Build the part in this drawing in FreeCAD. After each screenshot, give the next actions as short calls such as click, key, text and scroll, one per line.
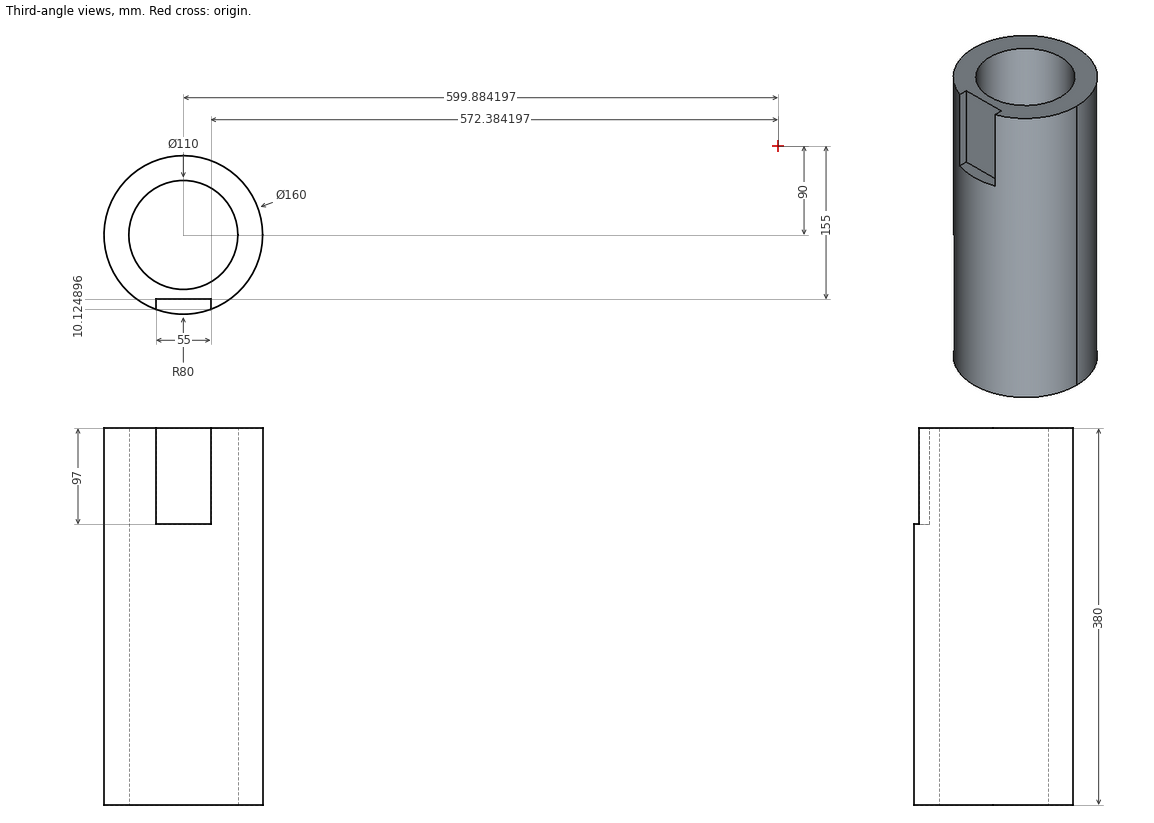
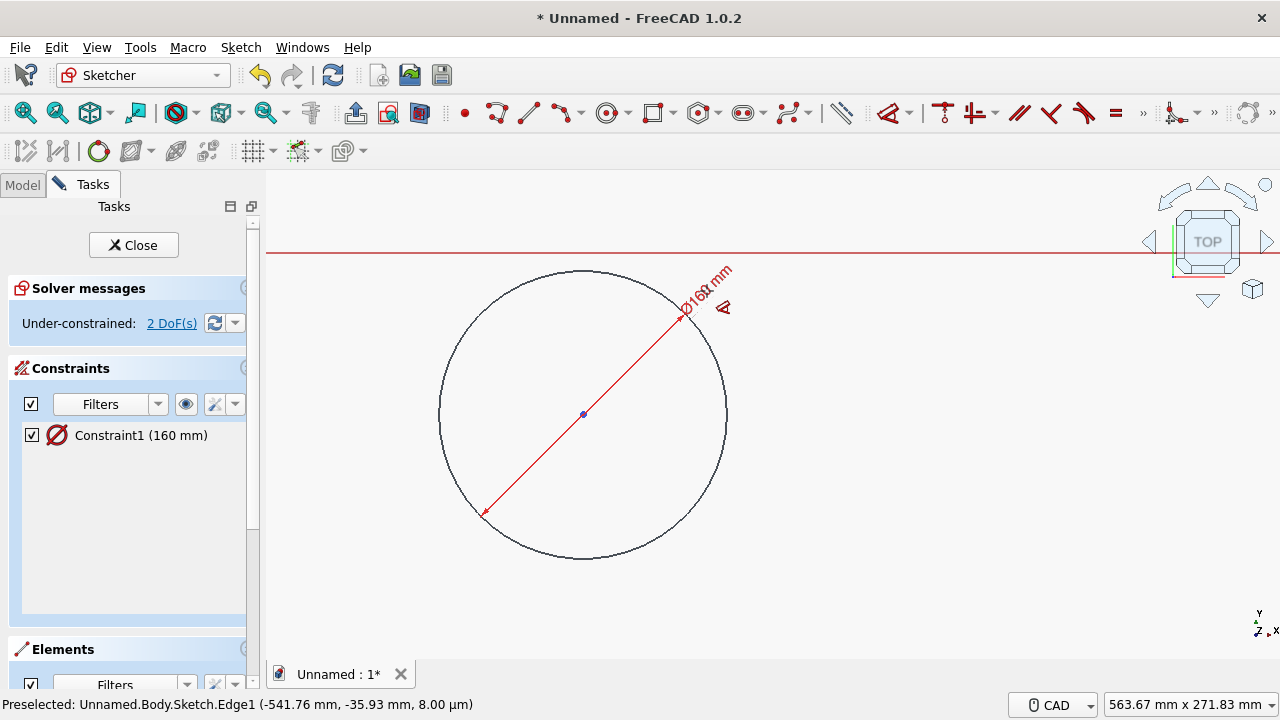
click(583, 415)
click(549, 334)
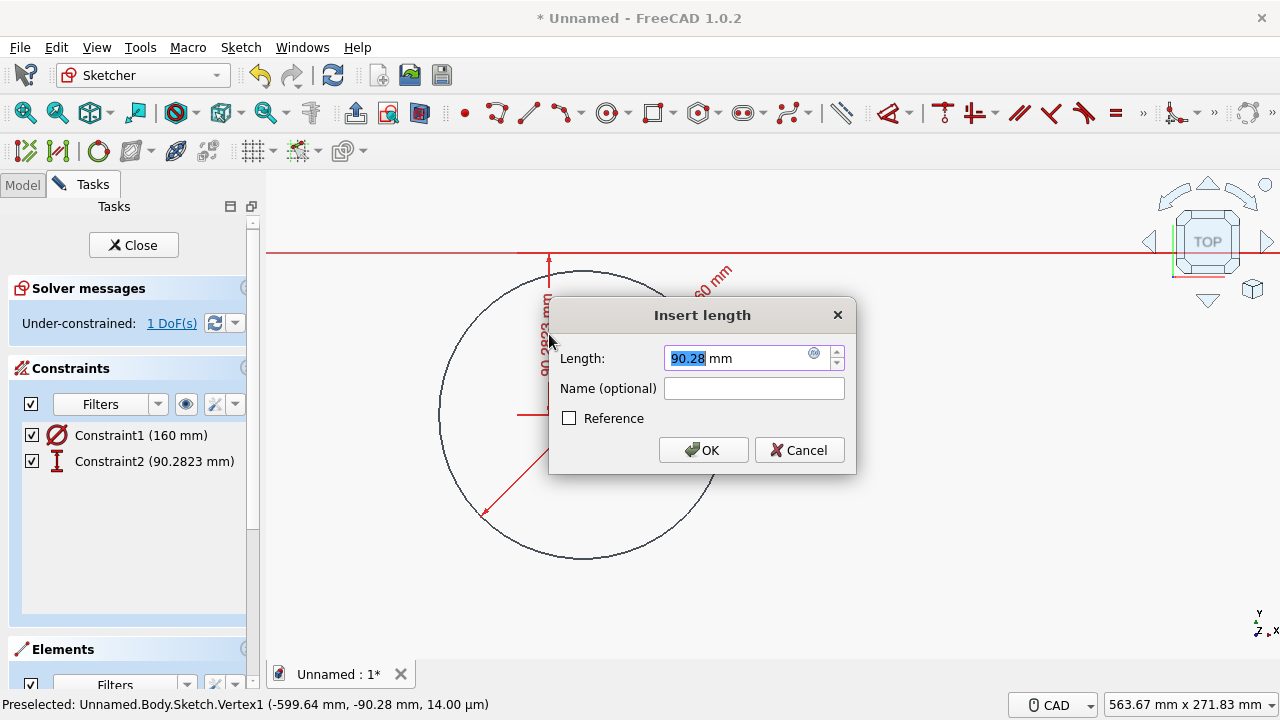
text(90)
key(Return)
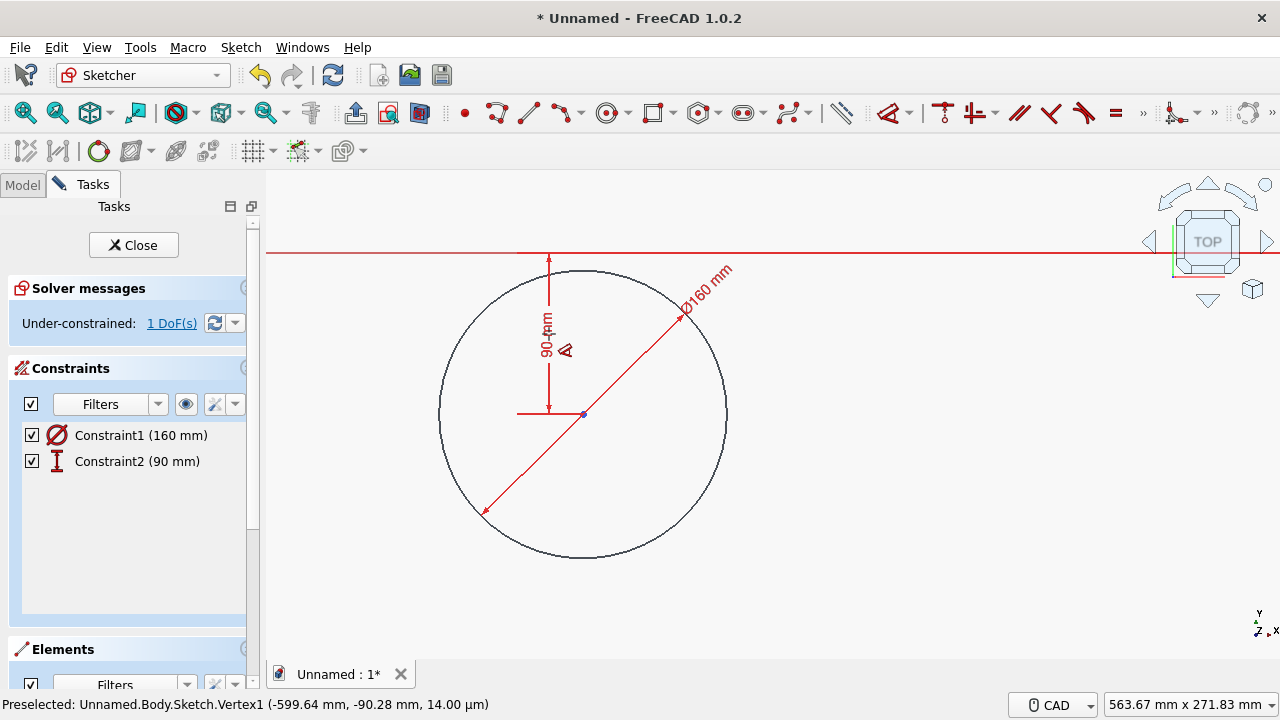
click(583, 414)
click(849, 219)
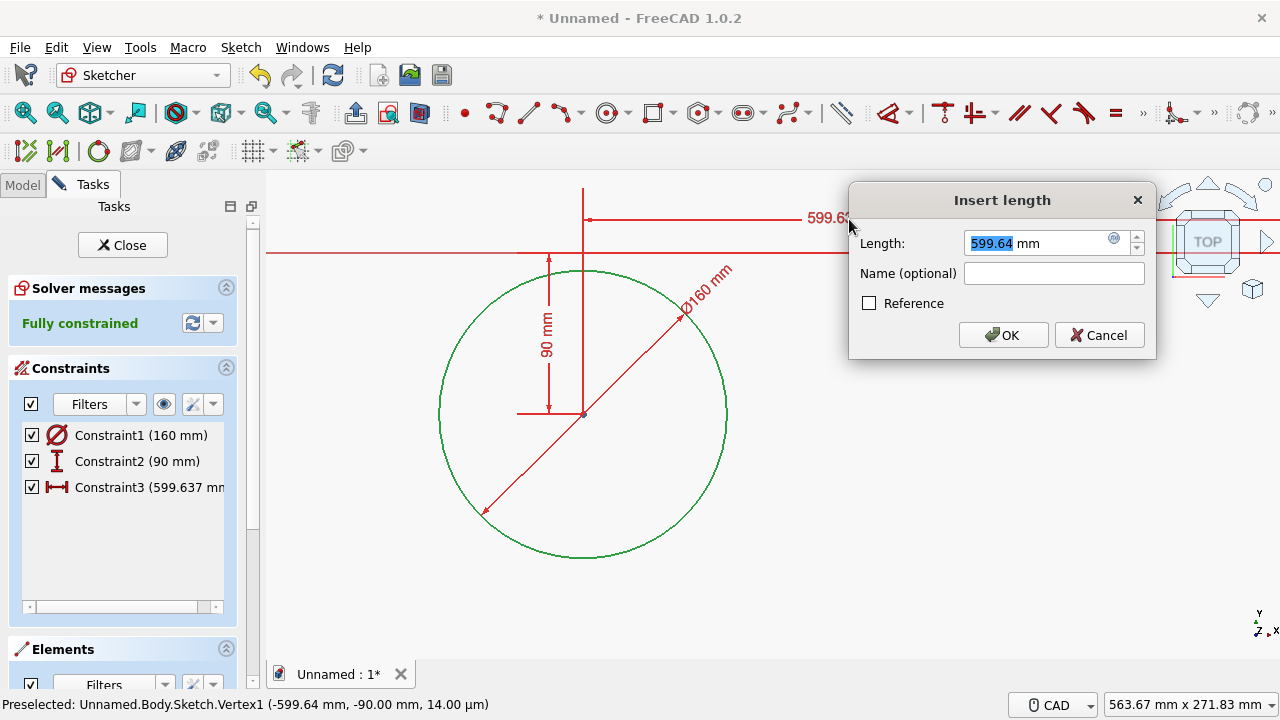
text(599.884197)
key(Return)
key(Escape)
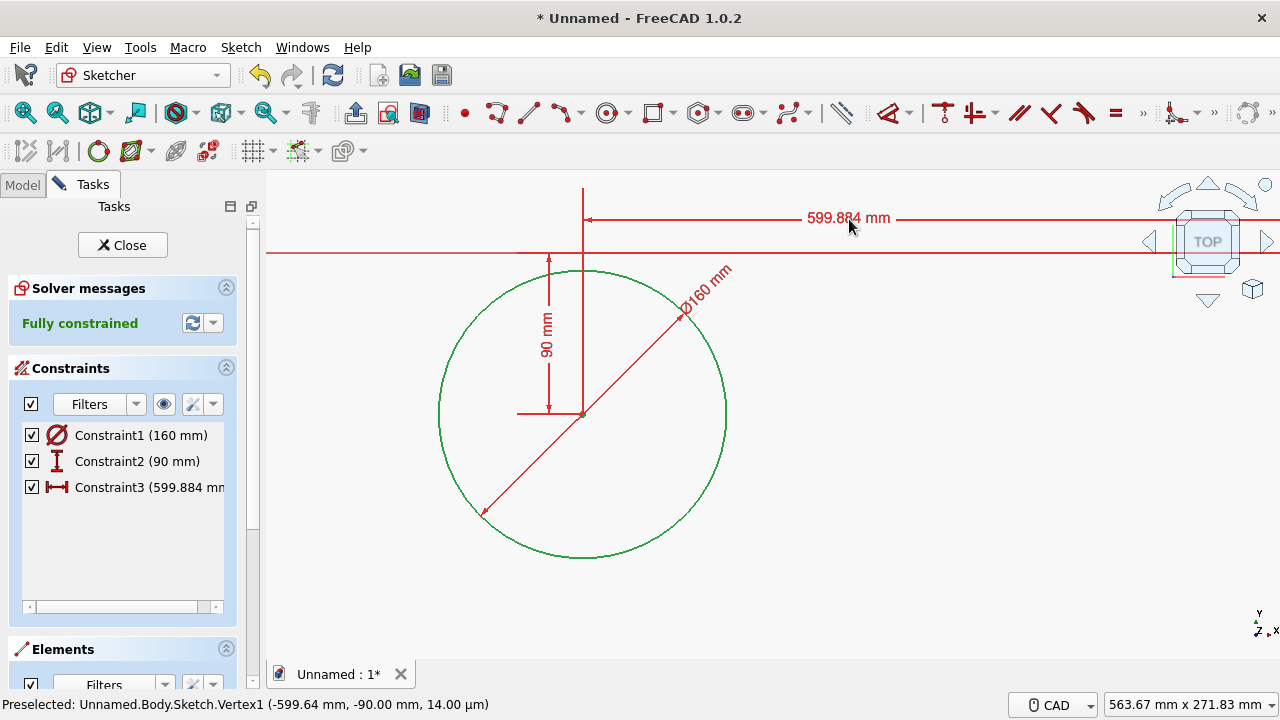
click(123, 245)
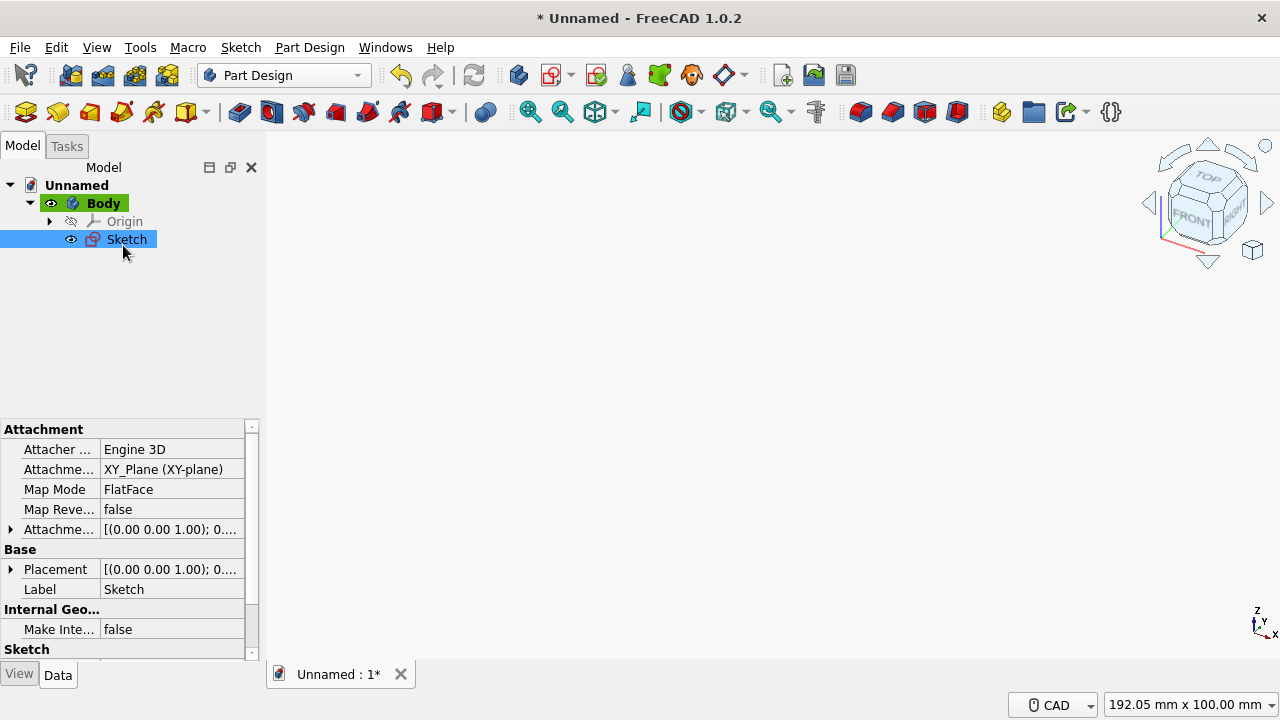
click(26, 112)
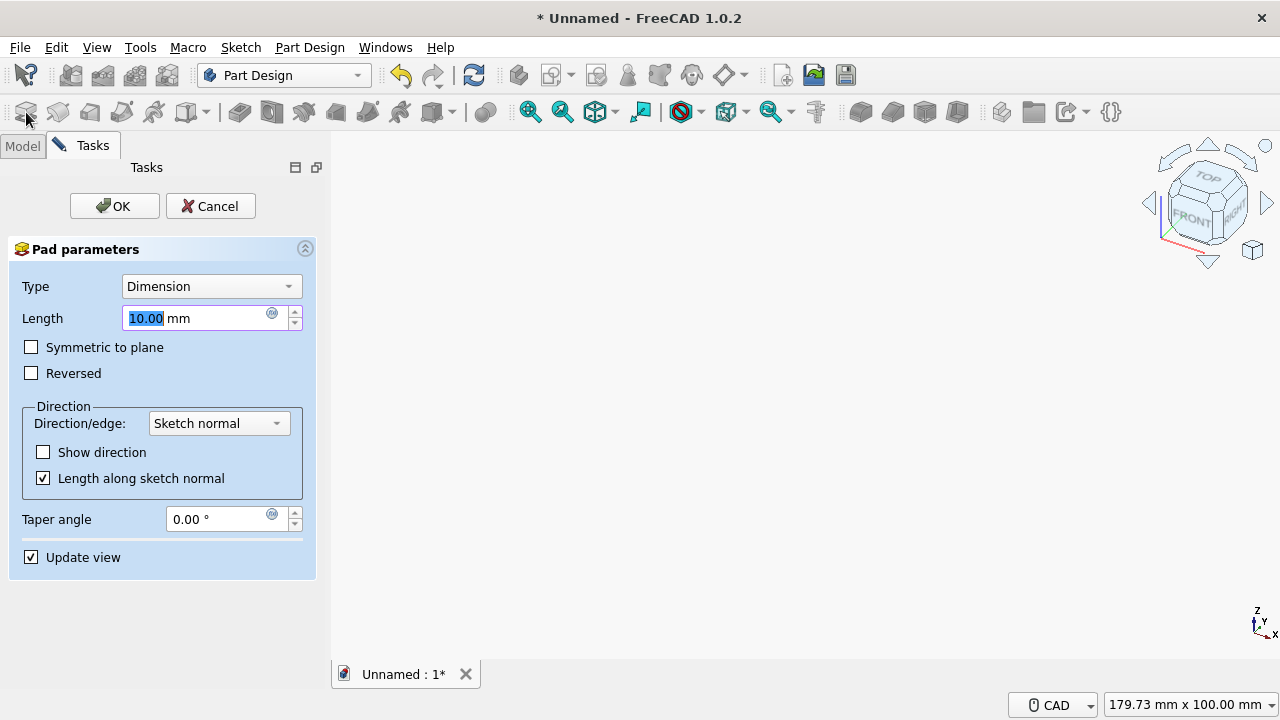
text(380)
key(Tab)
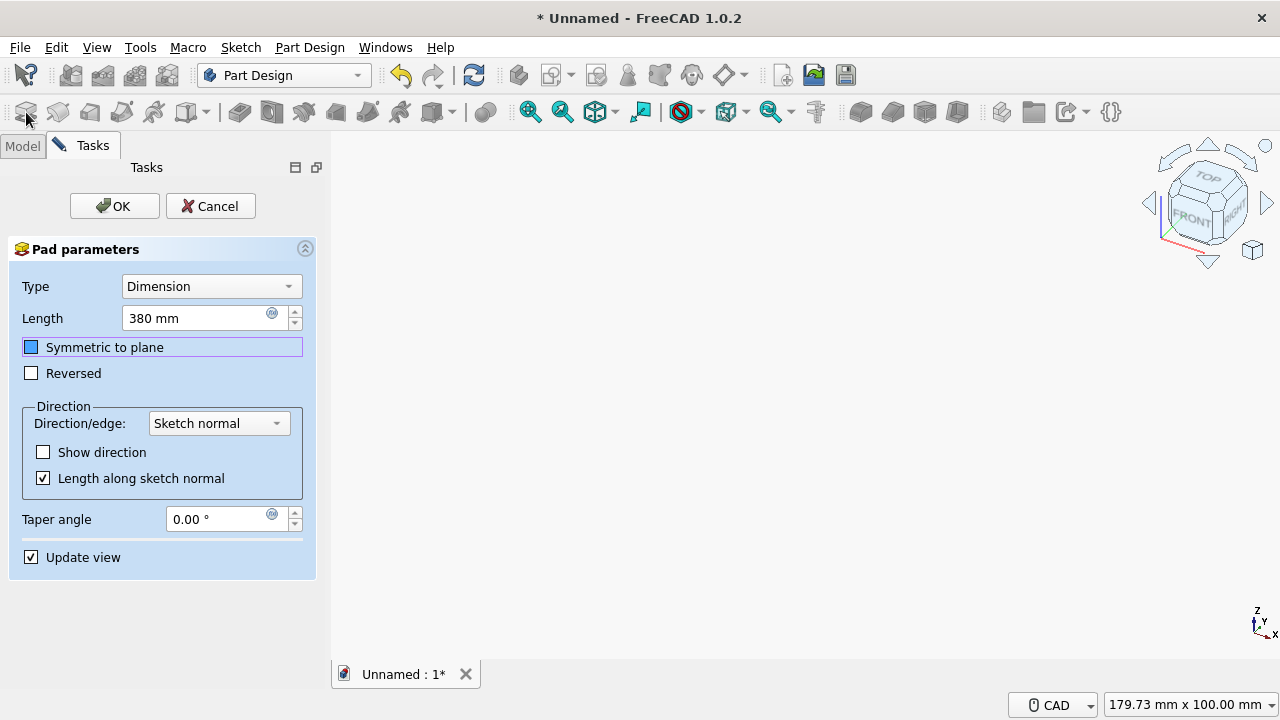
click(115, 206)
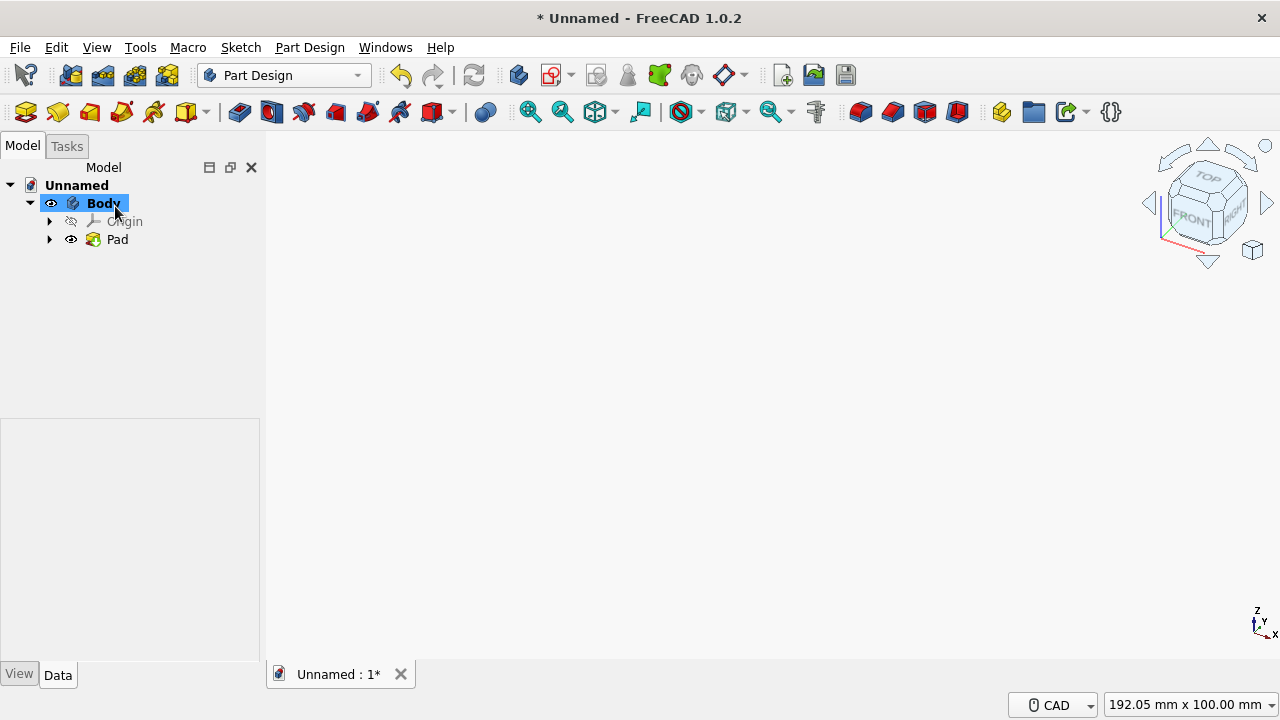
click(532, 112)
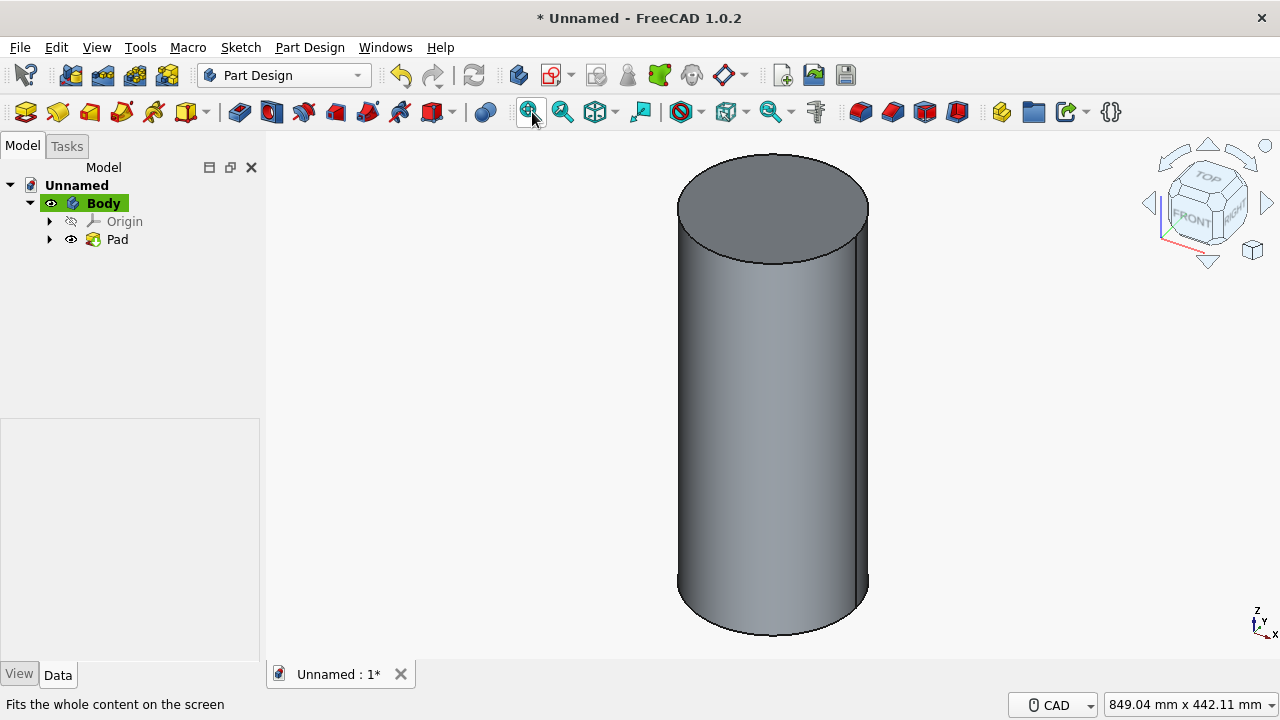
click(50, 221)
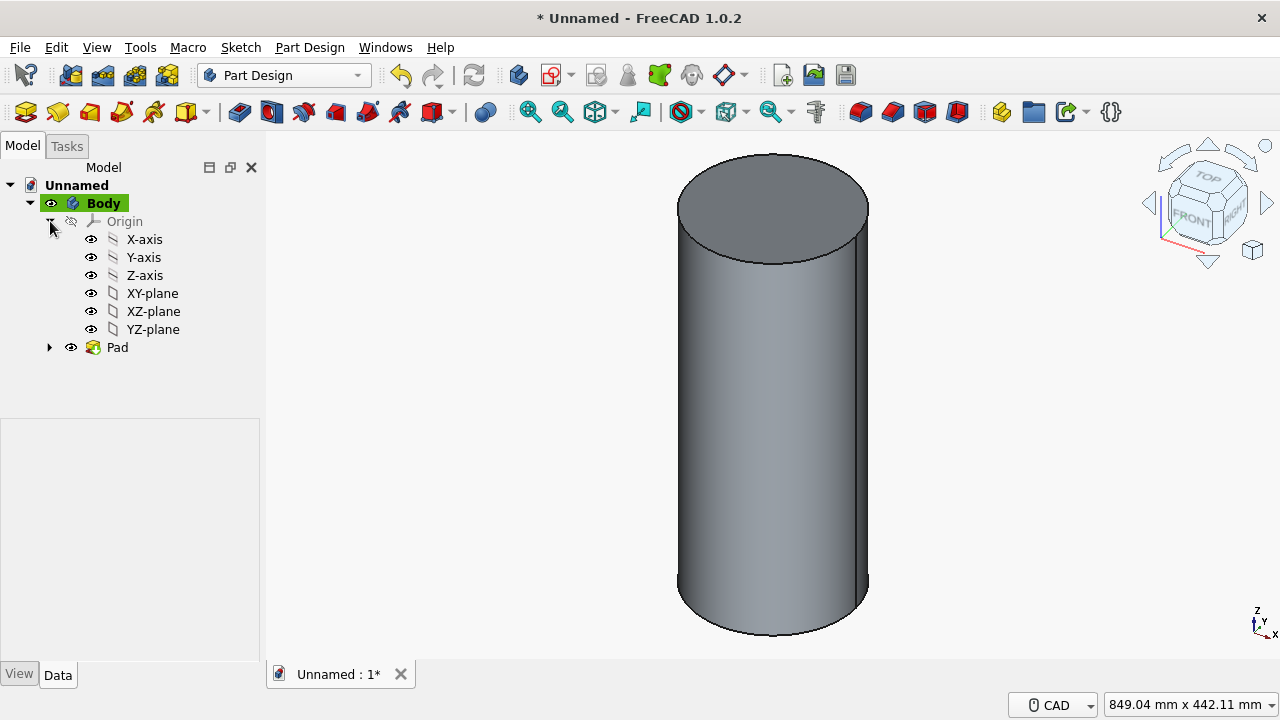
click(136, 293)